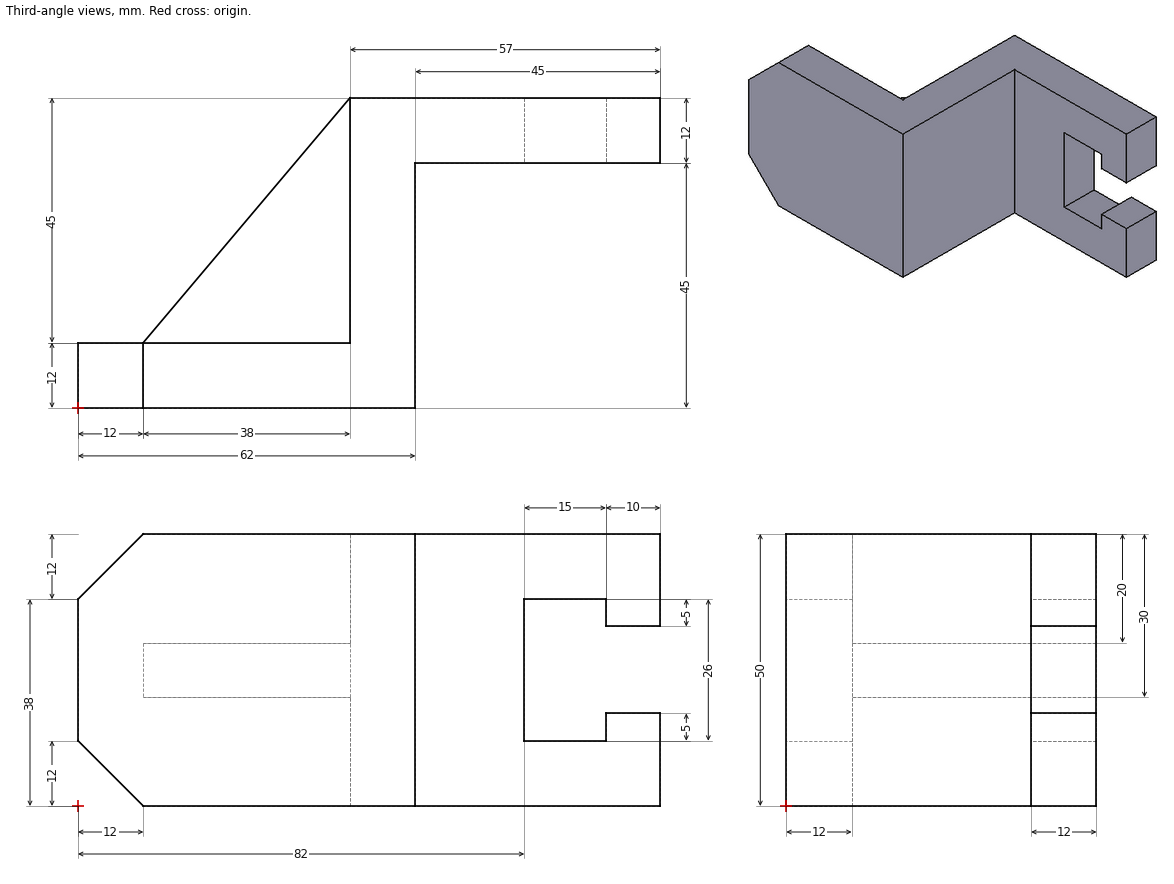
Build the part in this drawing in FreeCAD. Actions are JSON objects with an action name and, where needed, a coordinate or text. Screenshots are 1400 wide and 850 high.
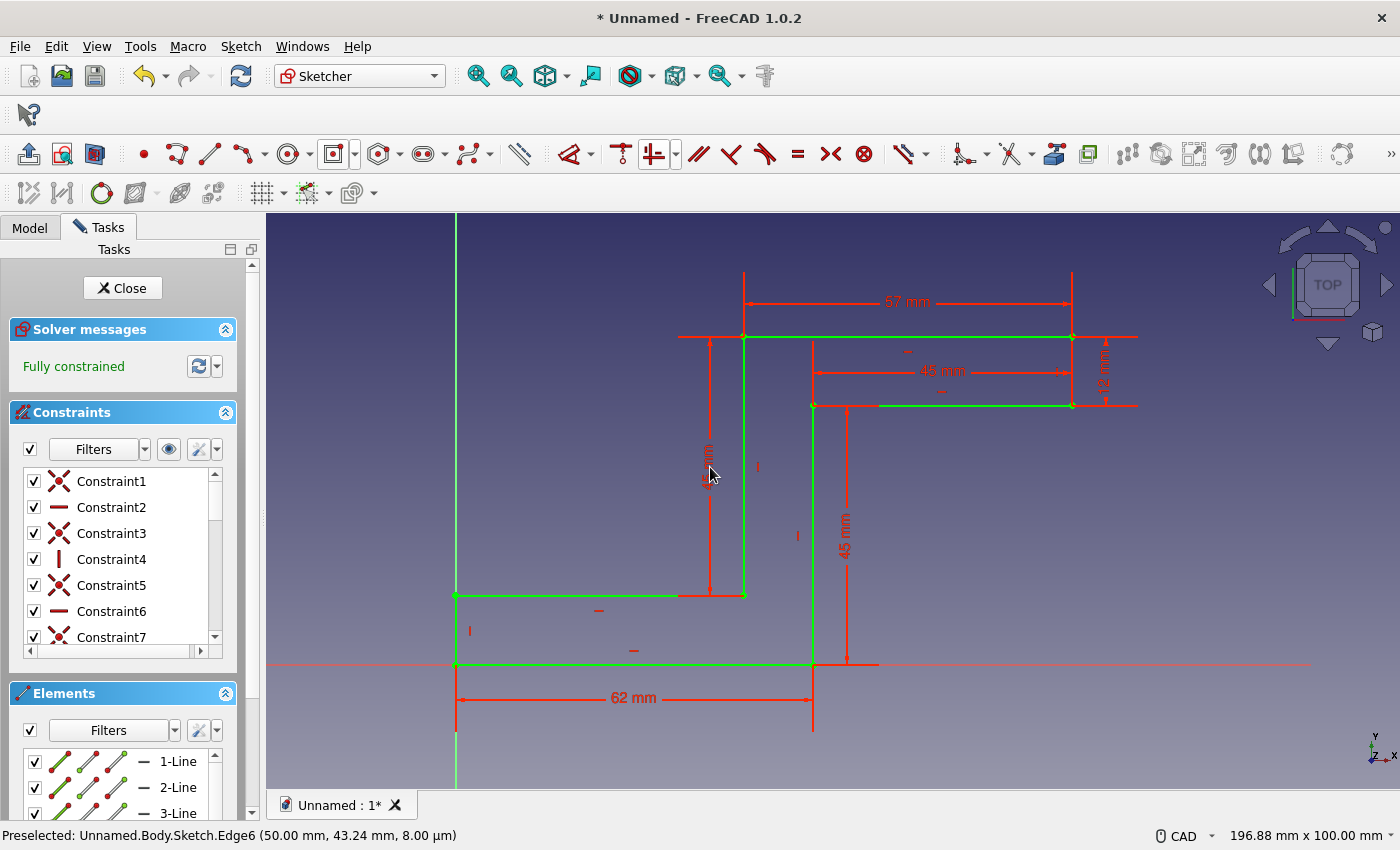
{"action": "left_click", "coordinate": [123, 288]}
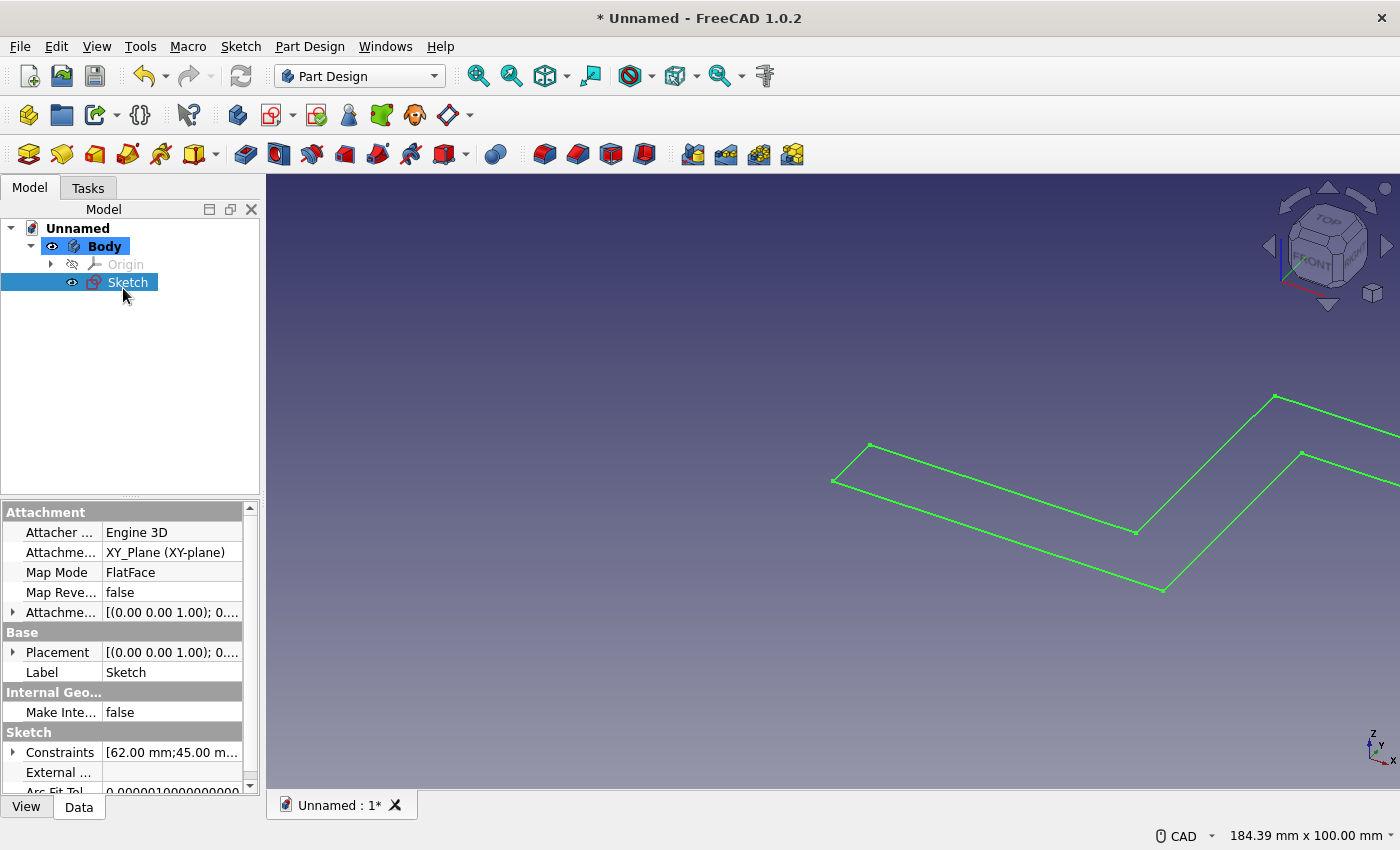
{"action": "left_click", "coordinate": [29, 154]}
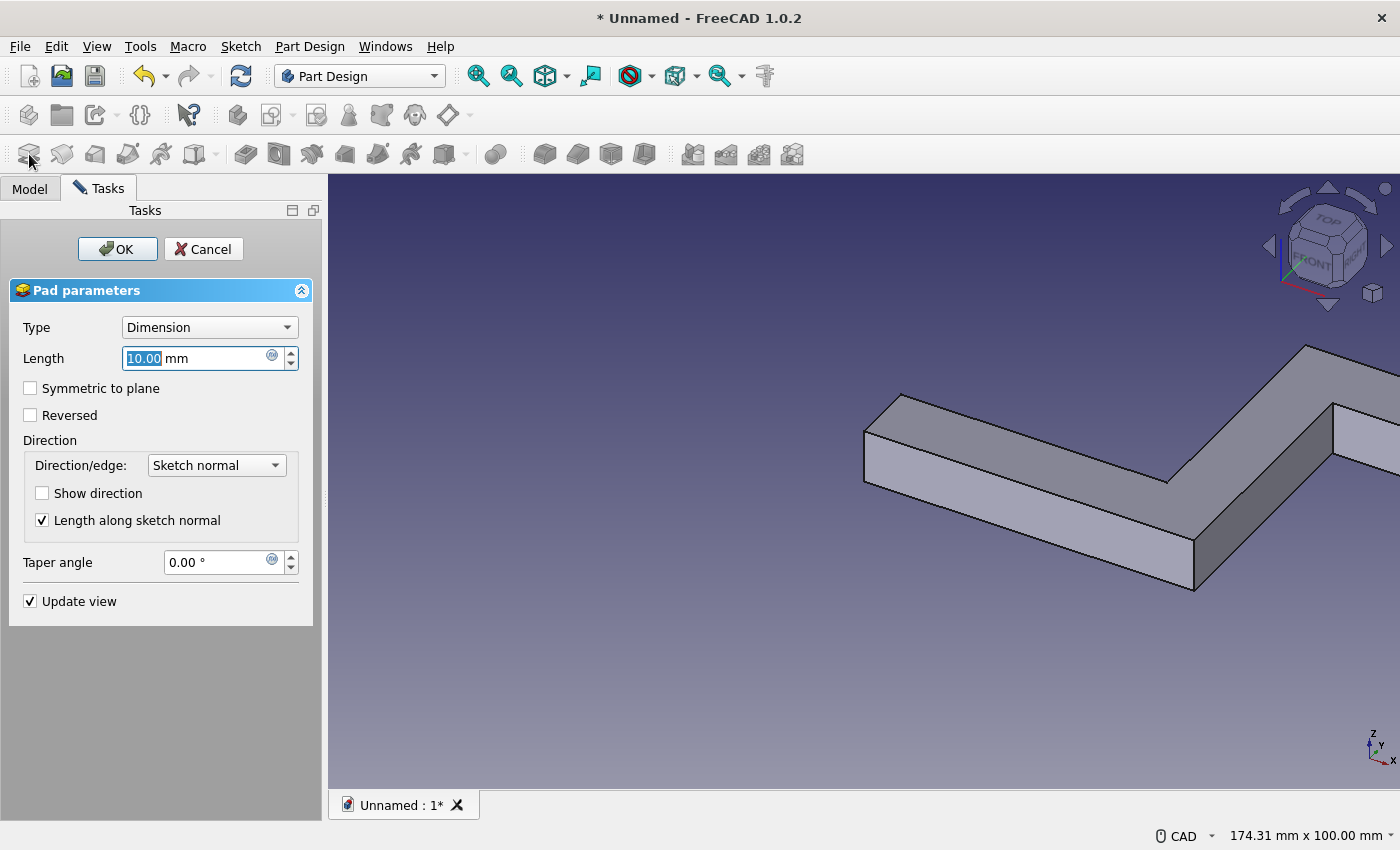
{"action": "type", "text": "50"}
{"action": "key", "text": "Tab"}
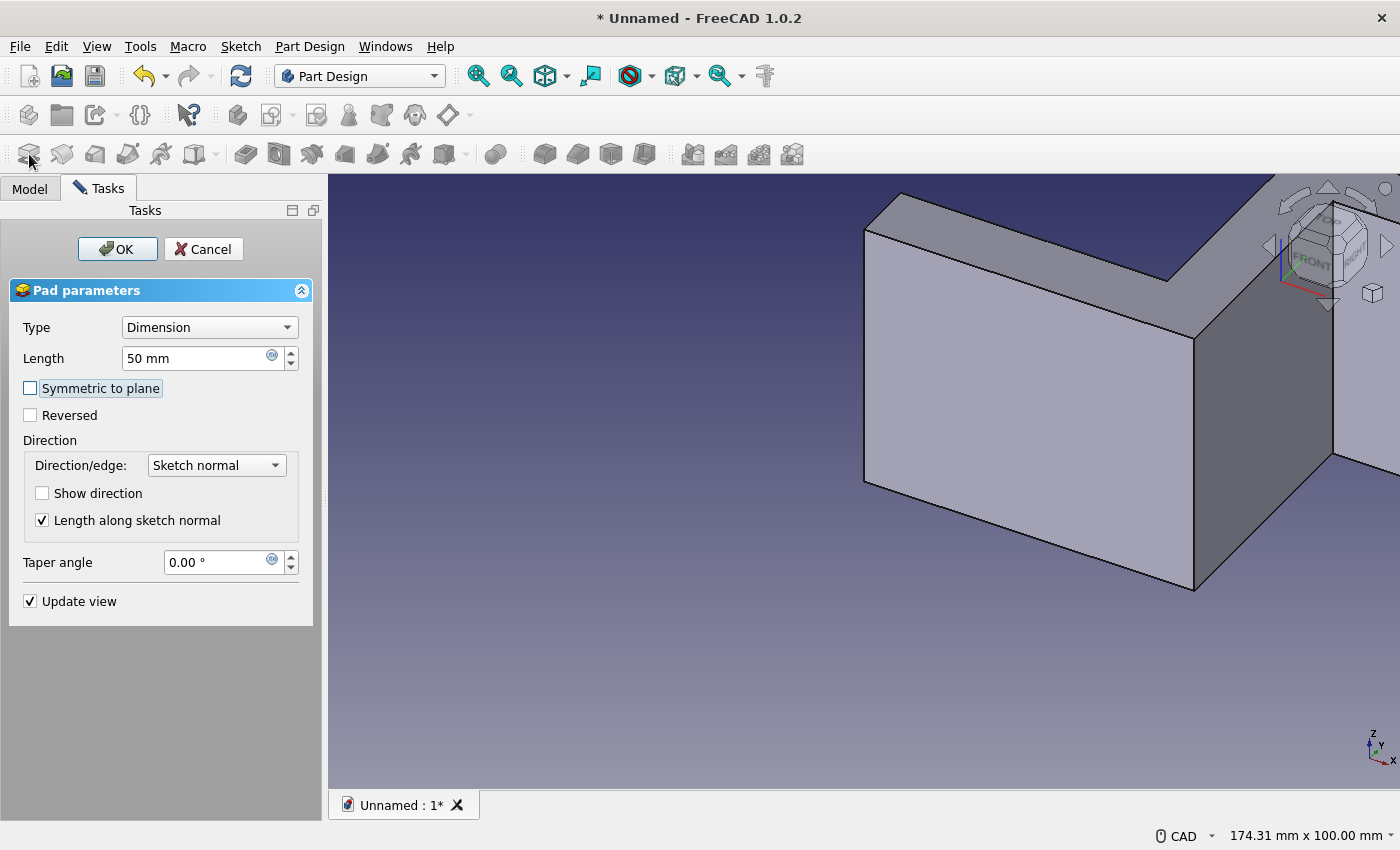
{"action": "left_click", "coordinate": [118, 249]}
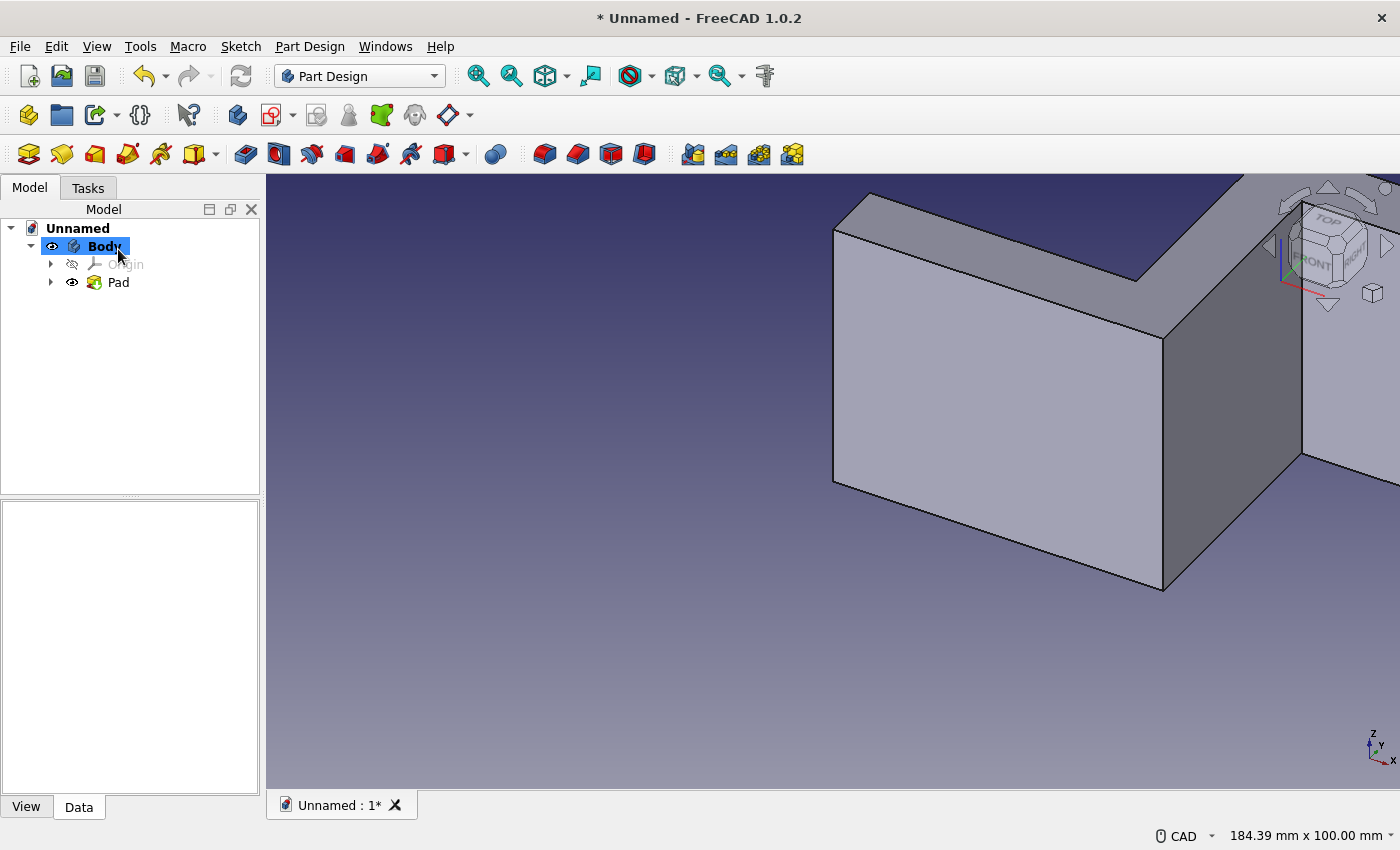
{"action": "left_click", "coordinate": [479, 76]}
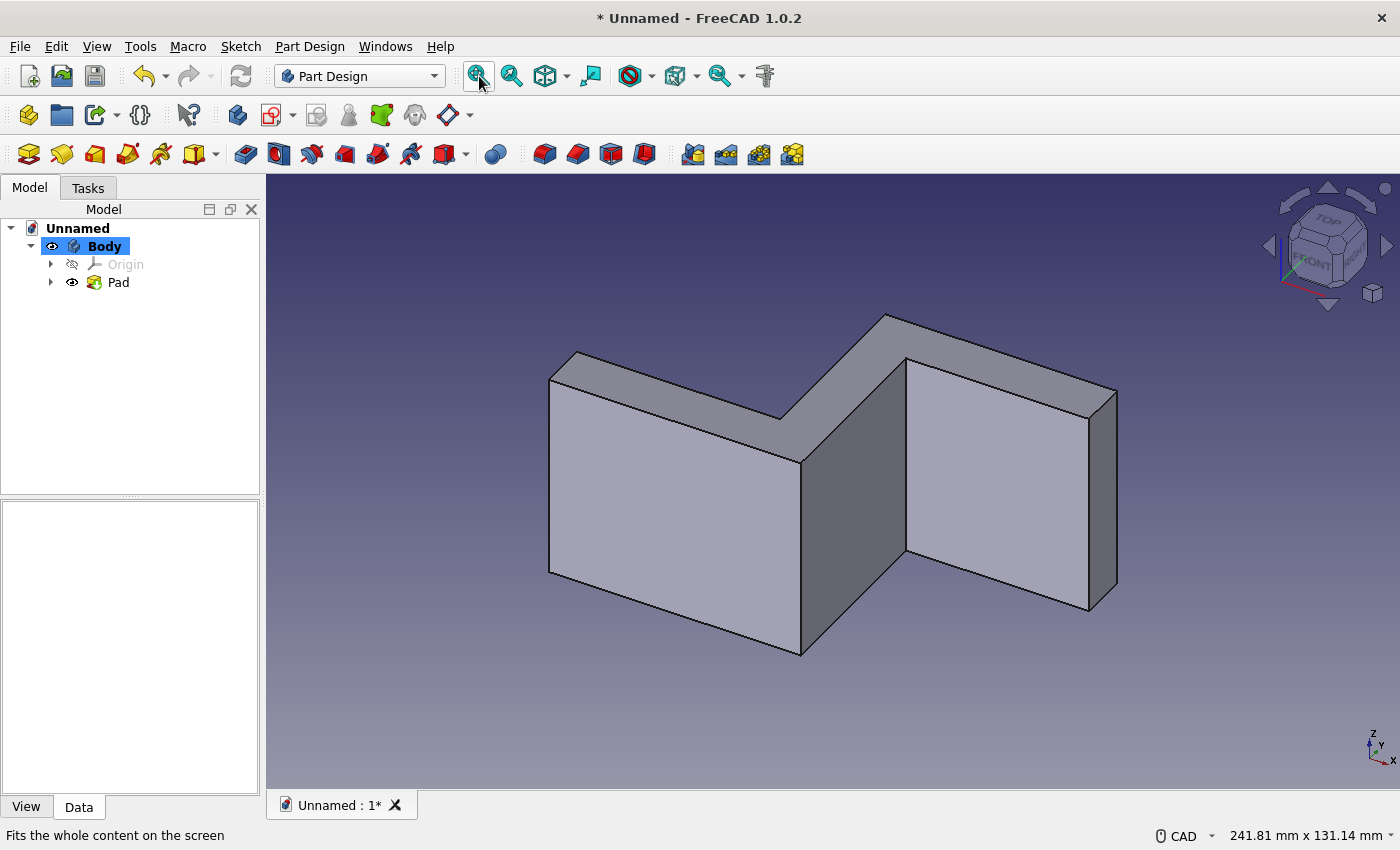
{"action": "key", "text": "4"}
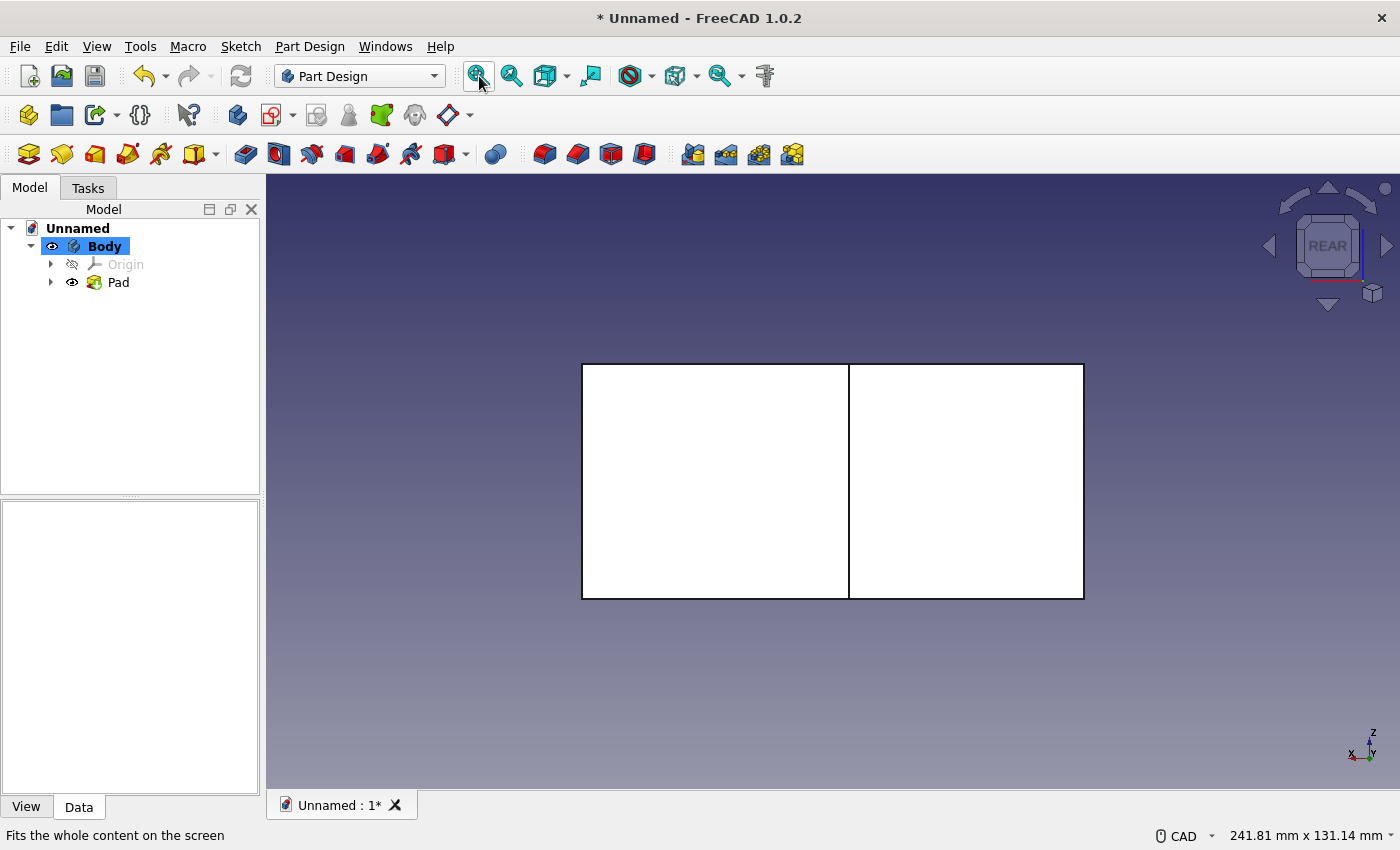
{"action": "left_click", "coordinate": [479, 76]}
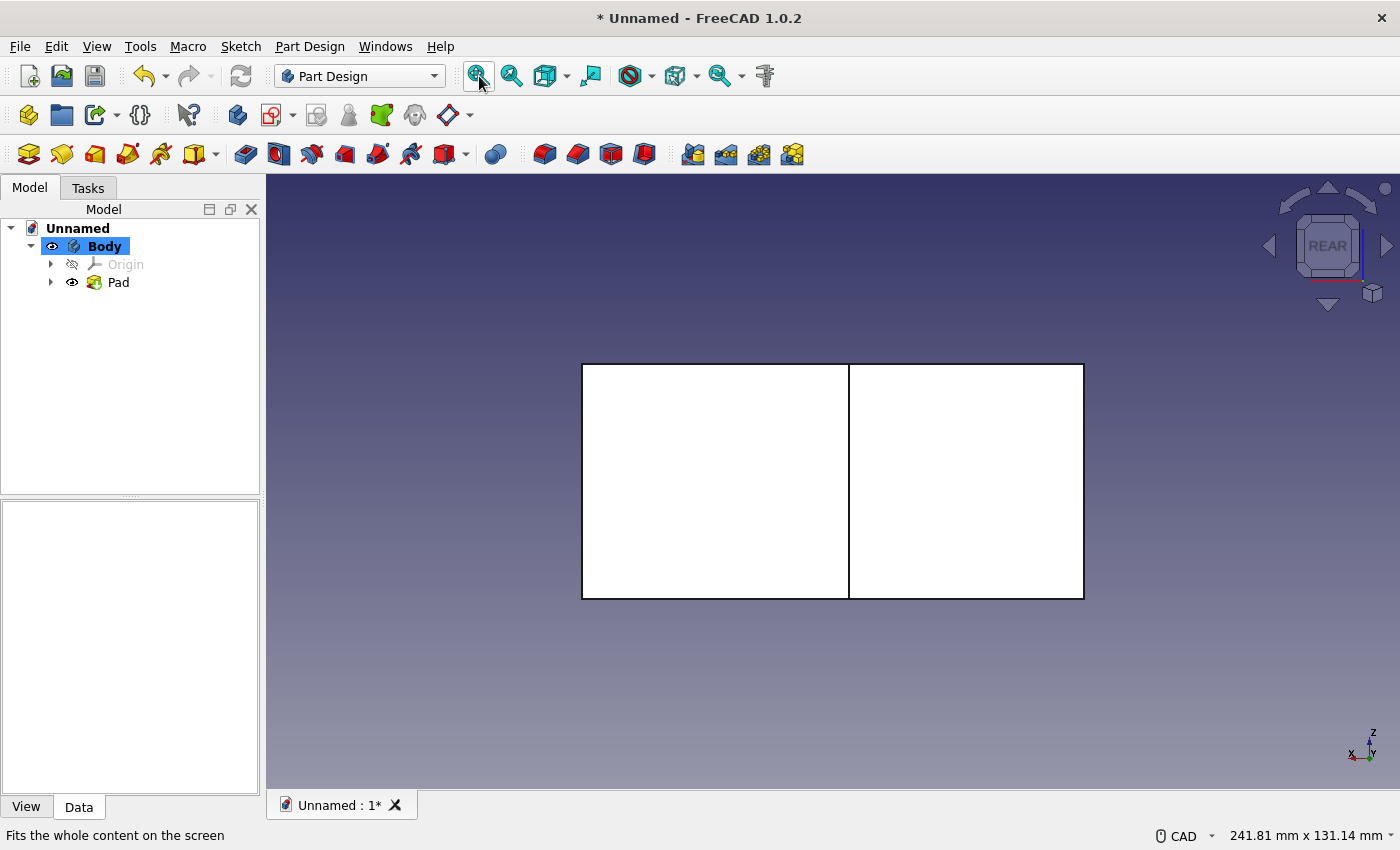
{"action": "left_click", "coordinate": [967, 481]}